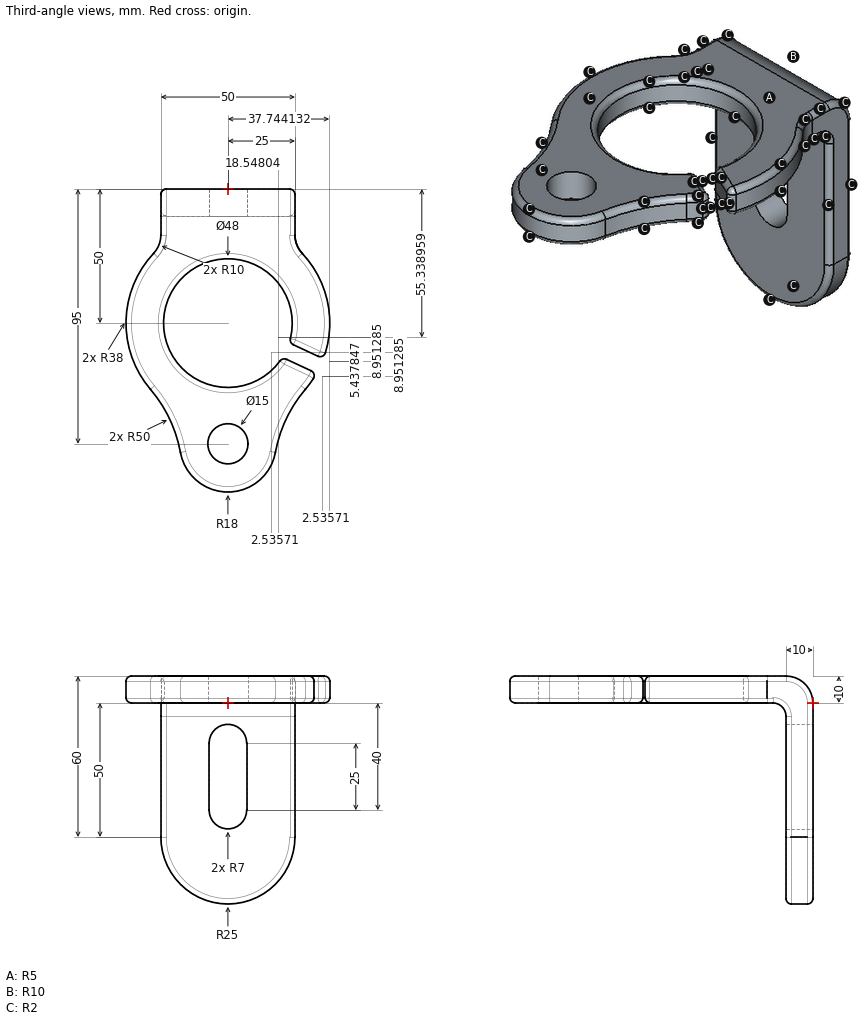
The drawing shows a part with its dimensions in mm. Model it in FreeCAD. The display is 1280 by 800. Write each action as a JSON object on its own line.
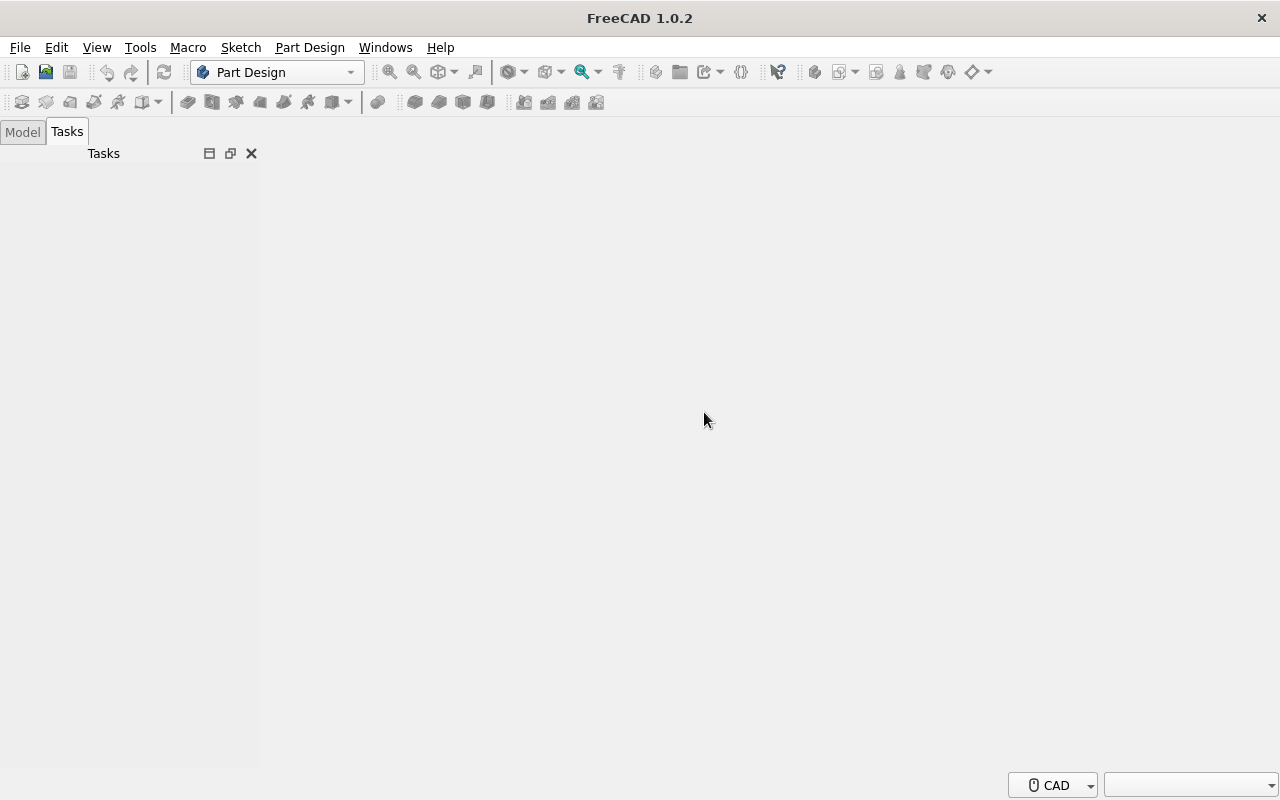
{"action": "left_click", "coordinate": [22, 72]}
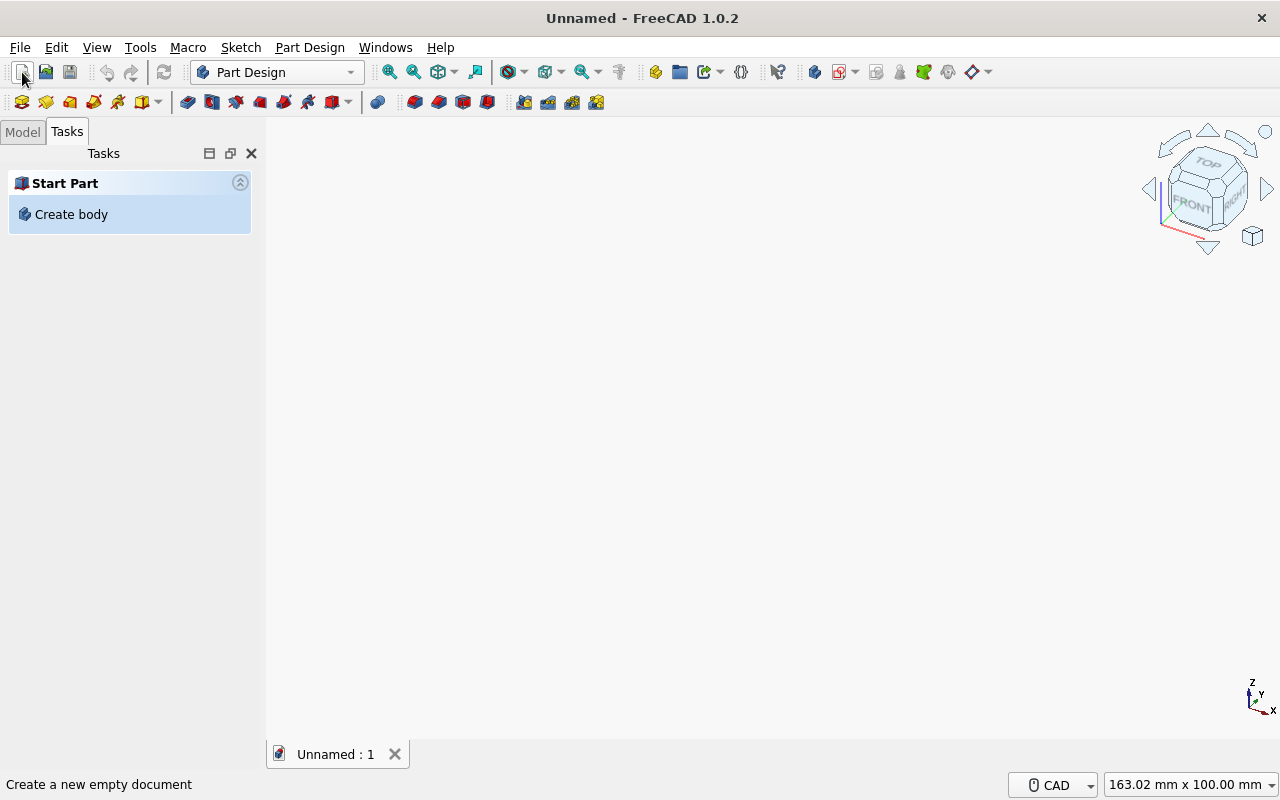
{"action": "left_click", "coordinate": [840, 72]}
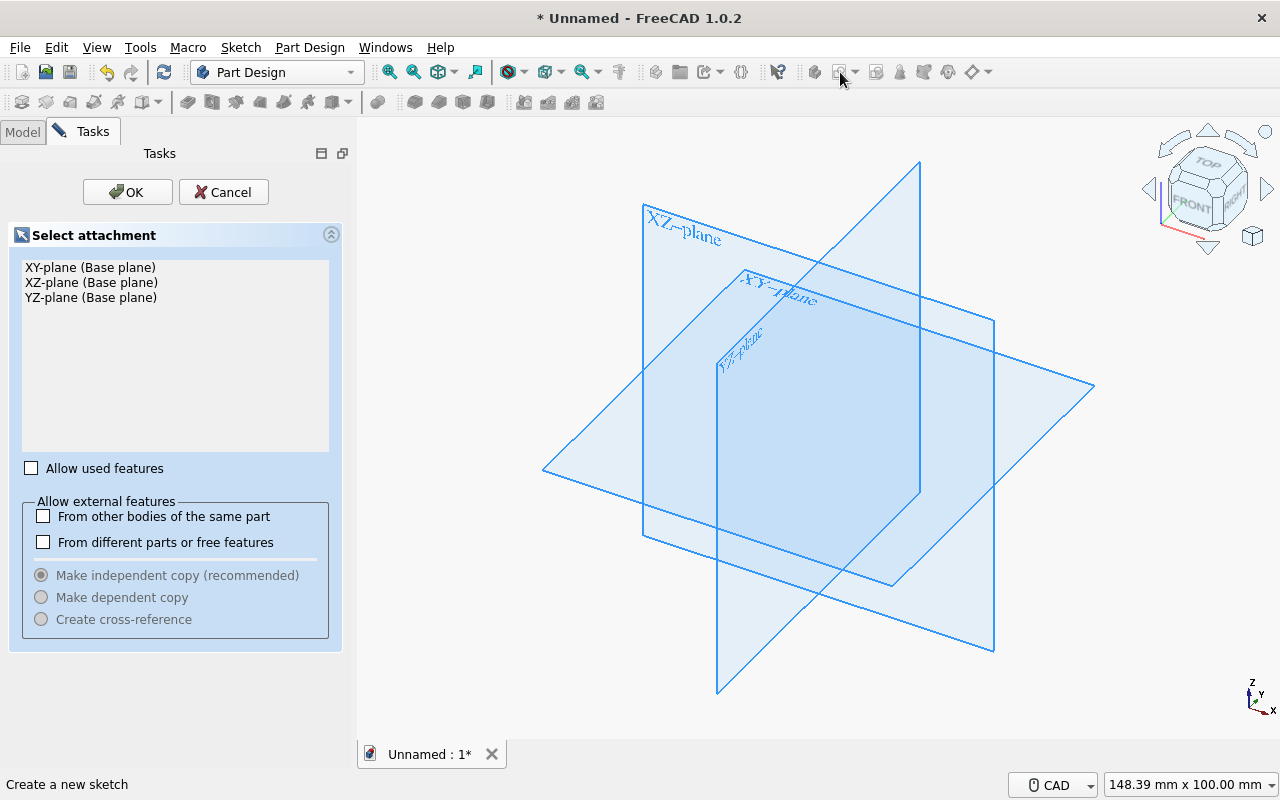
{"action": "left_click", "coordinate": [82, 268]}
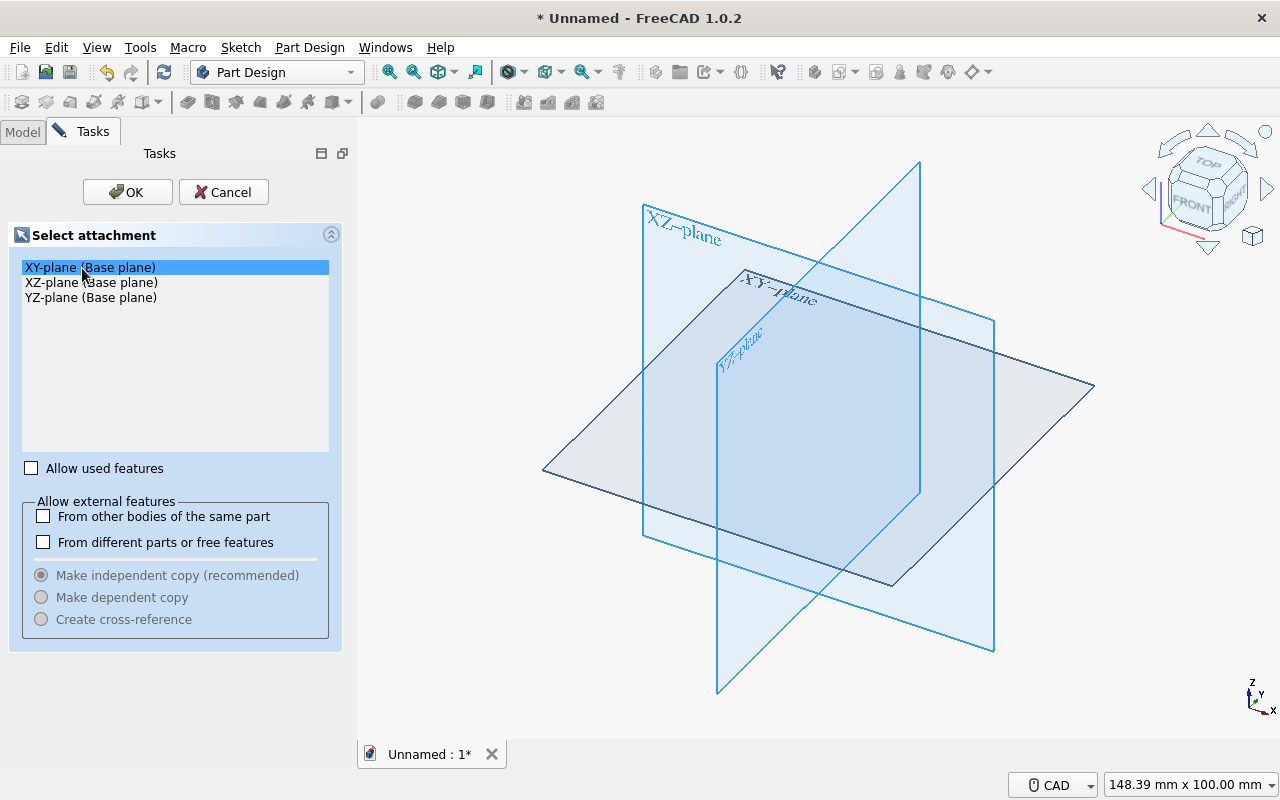
{"action": "left_click", "coordinate": [128, 192]}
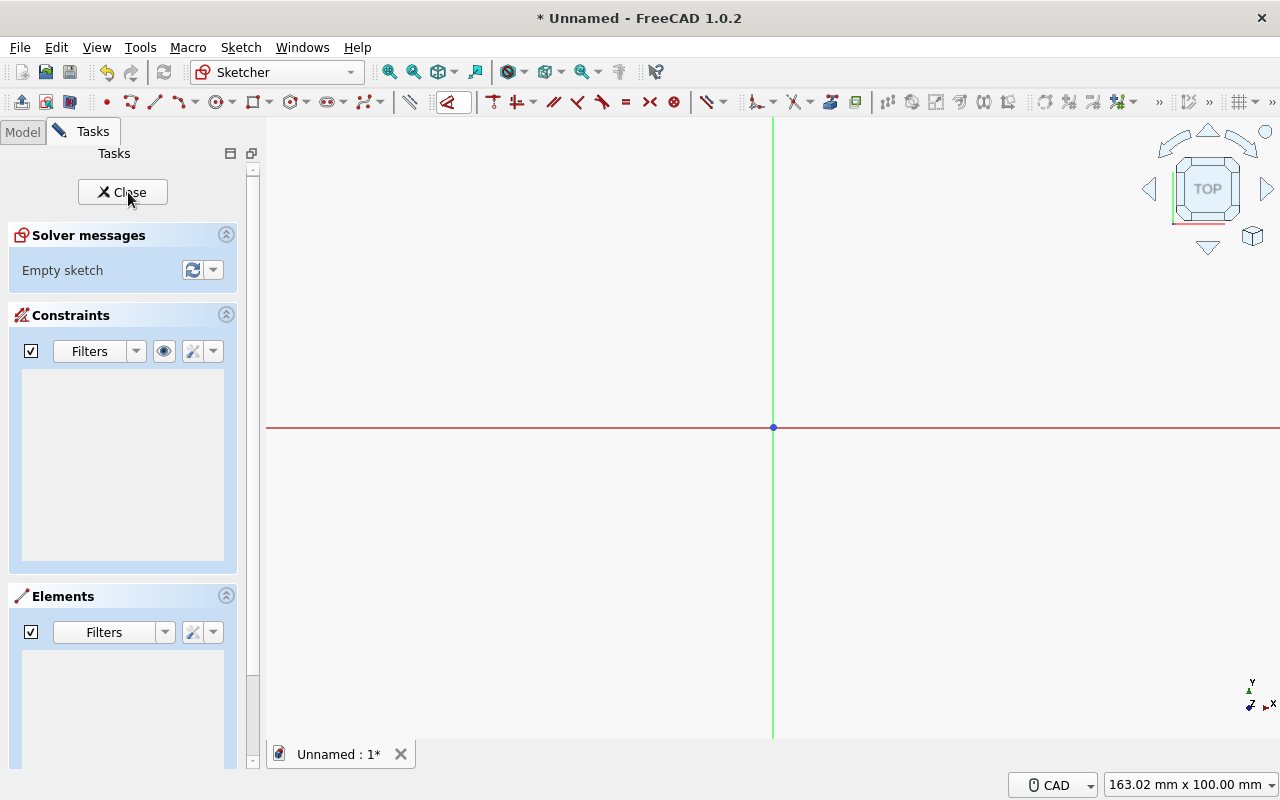
{"action": "scroll", "coordinate": [649, 145], "scroll_direction": "down", "scroll_amount": 4}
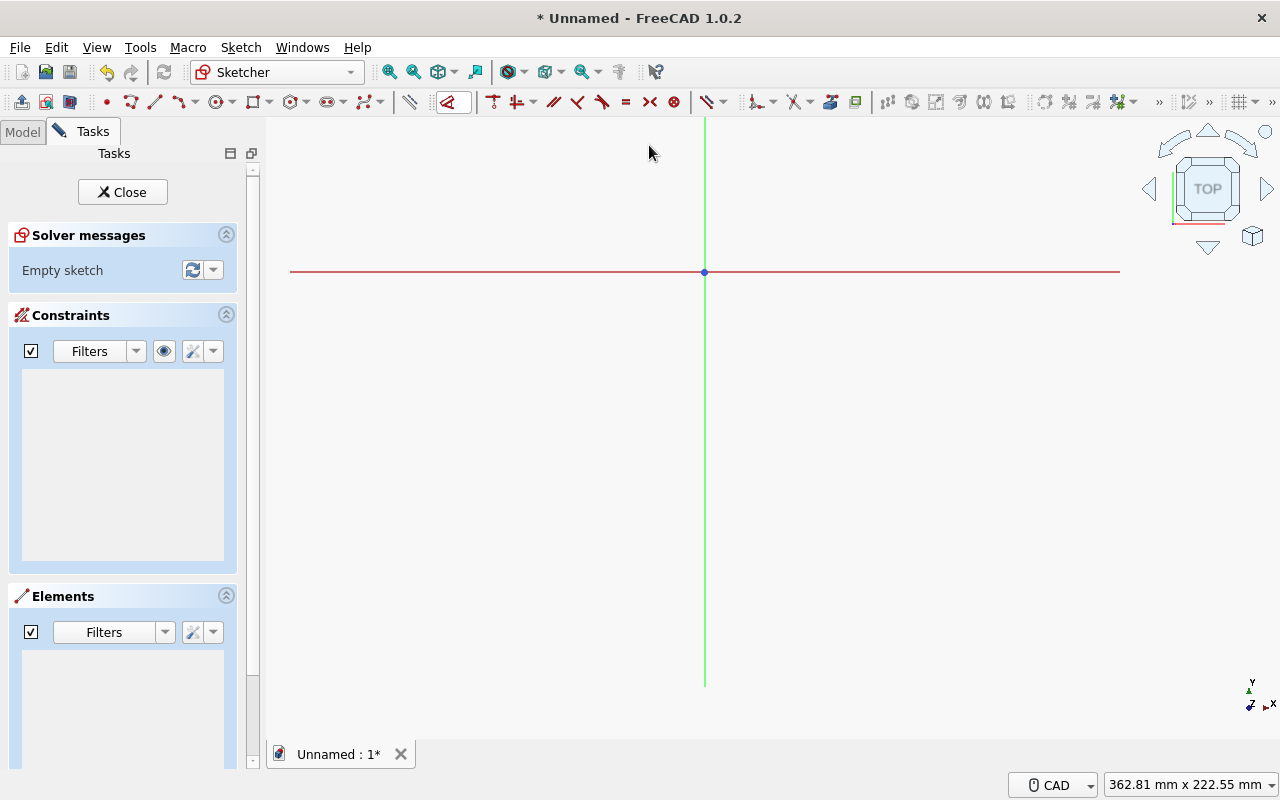
{"action": "left_click", "coordinate": [132, 102]}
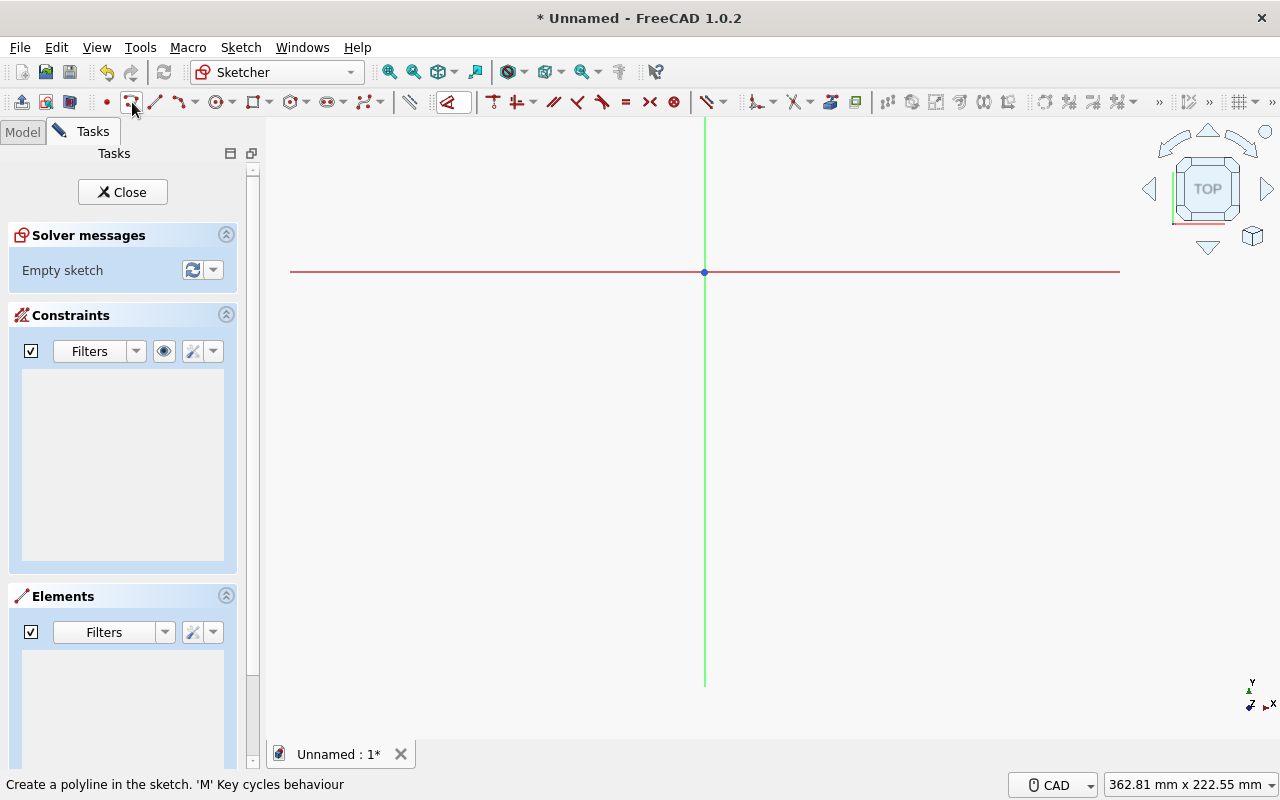
{"action": "left_click", "coordinate": [775, 320]}
{"action": "left_click", "coordinate": [775, 272]}
{"action": "left_click", "coordinate": [635, 281]}
{"action": "left_click", "coordinate": [635, 320]}
{"action": "right_click", "coordinate": [635, 320]}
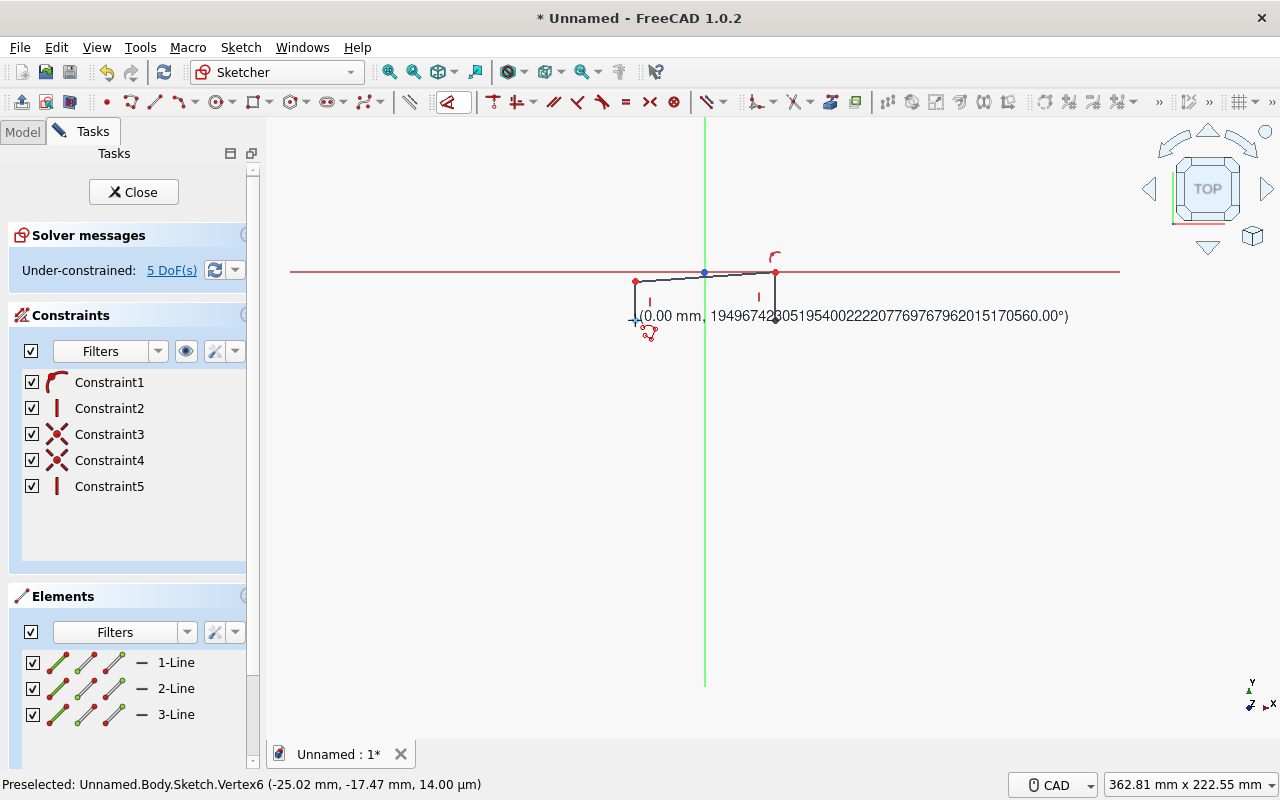
{"action": "left_click", "coordinate": [180, 102]}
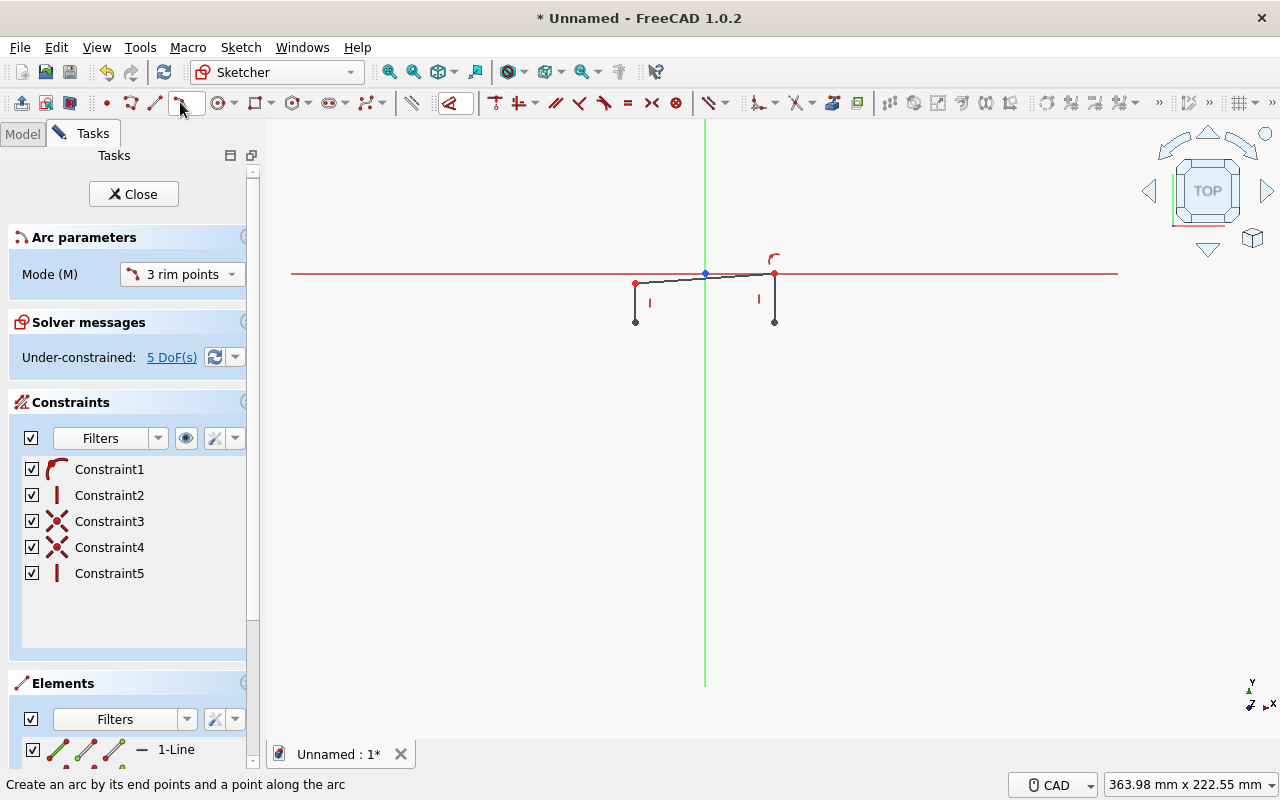
{"action": "left_click", "coordinate": [635, 322]}
{"action": "left_click", "coordinate": [628, 341]}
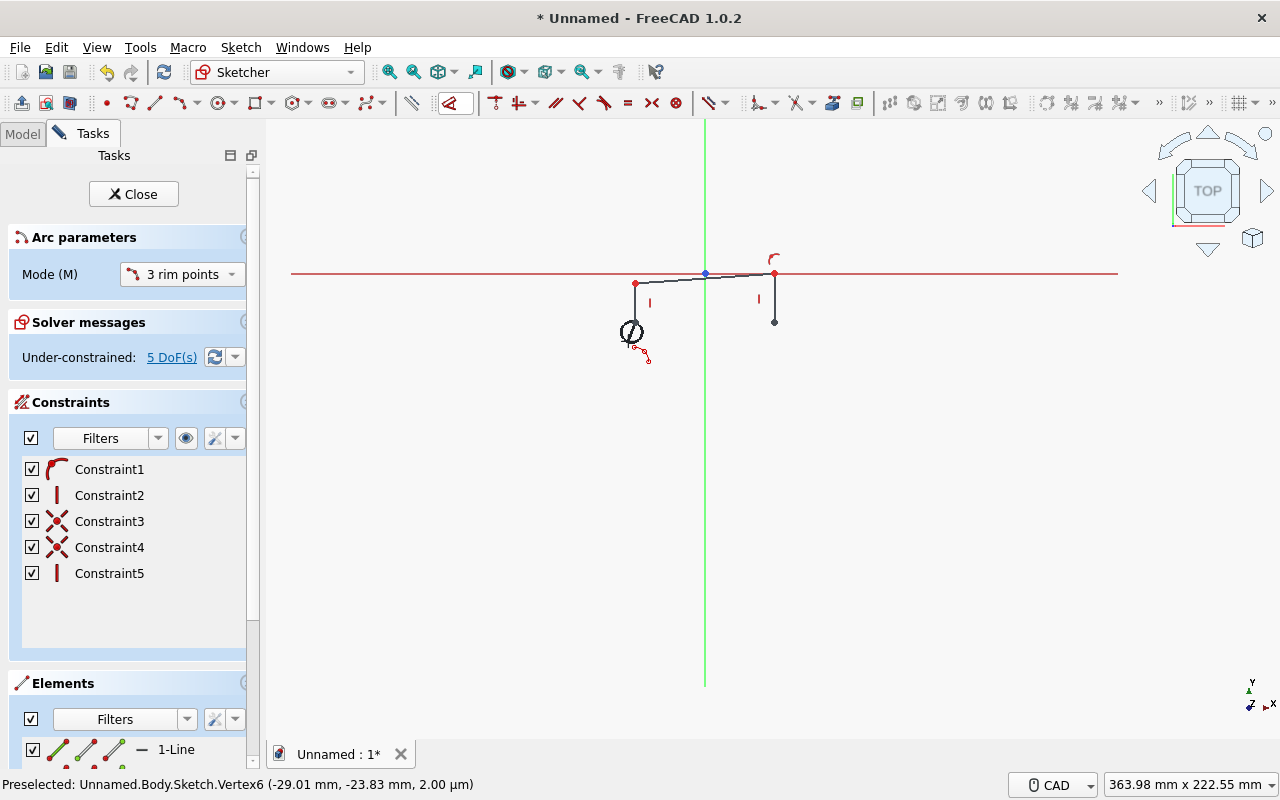
{"action": "scroll", "coordinate": [634, 332], "scroll_direction": "up", "scroll_amount": 11}